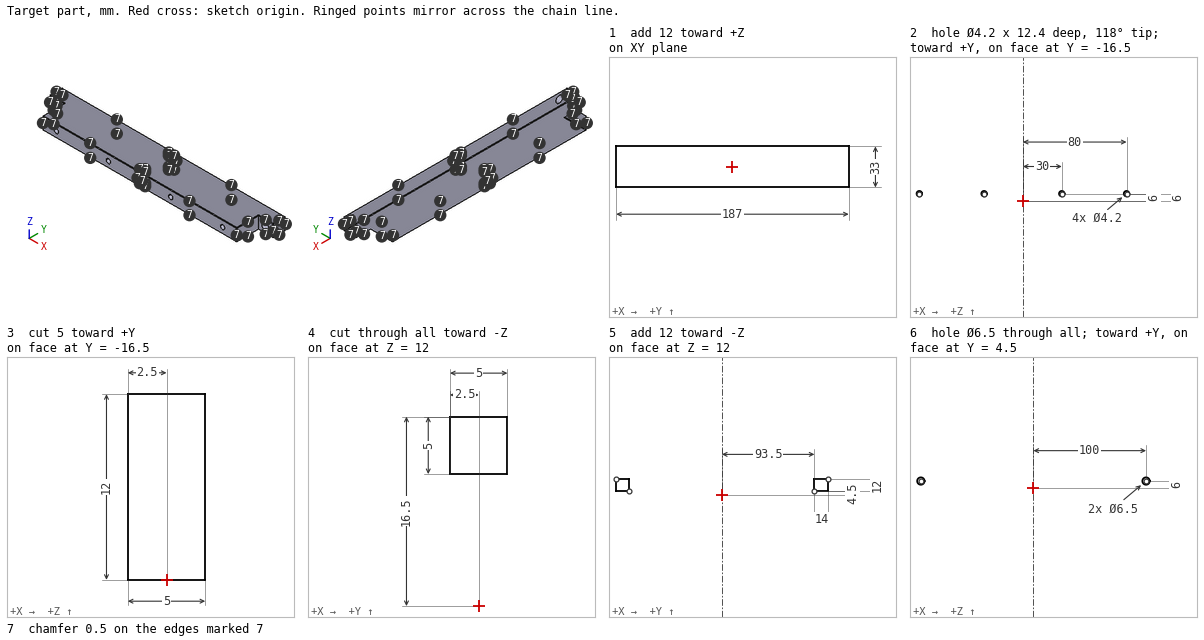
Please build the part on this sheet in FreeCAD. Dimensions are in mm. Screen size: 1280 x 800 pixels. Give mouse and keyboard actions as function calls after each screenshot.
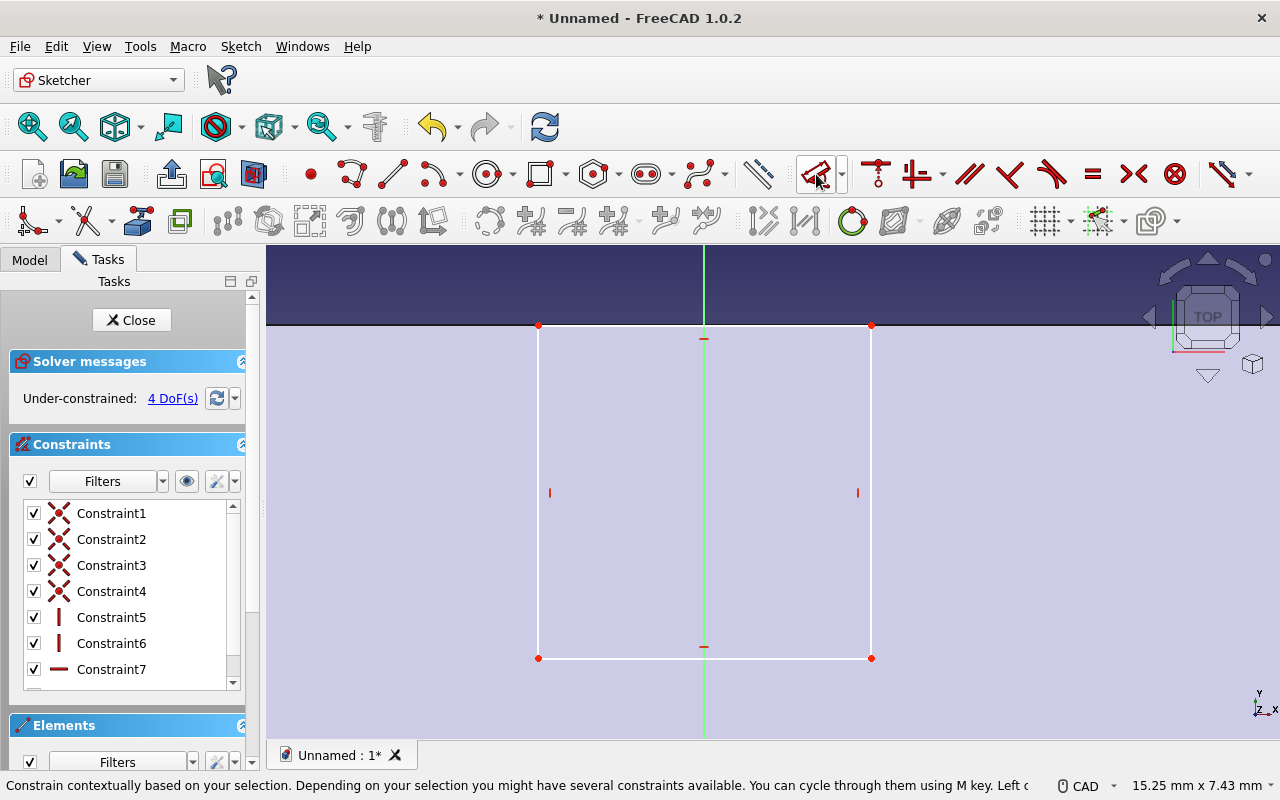
click(538, 426)
click(504, 493)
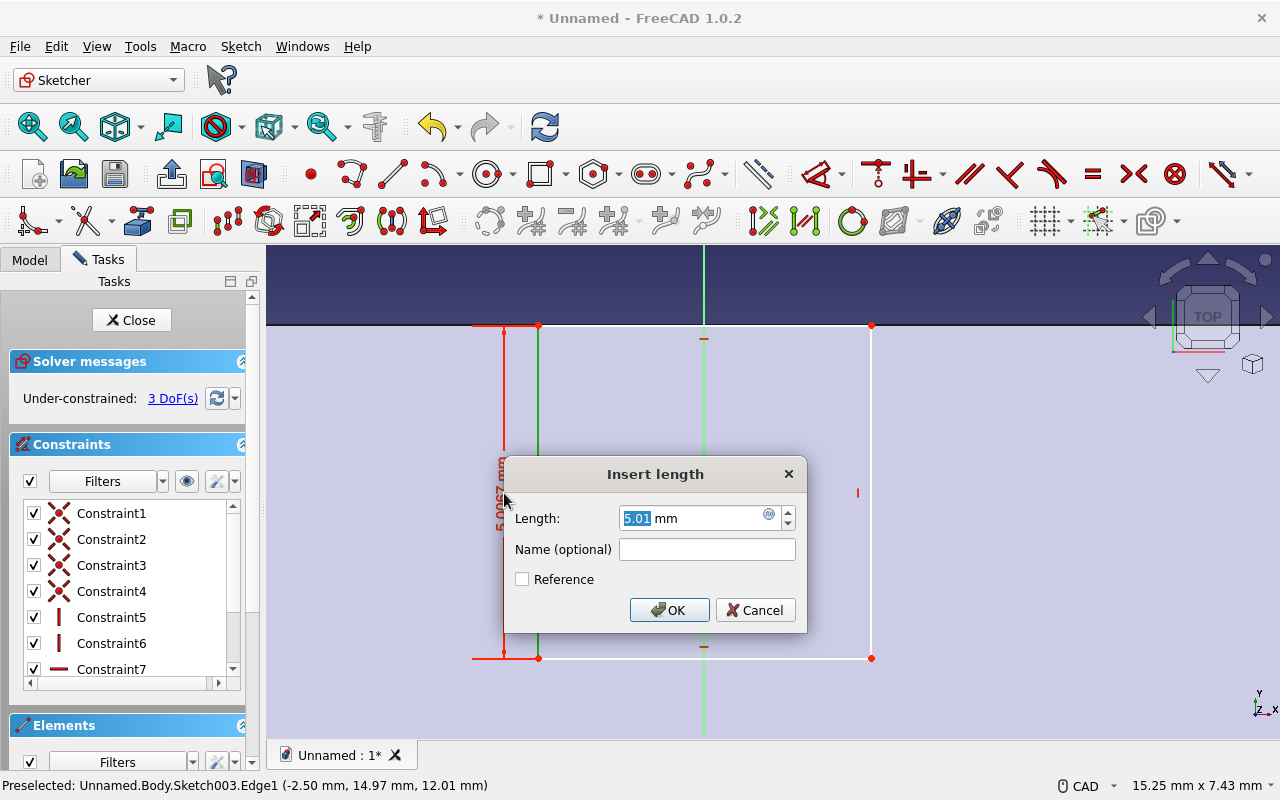
text(5)
key(Return)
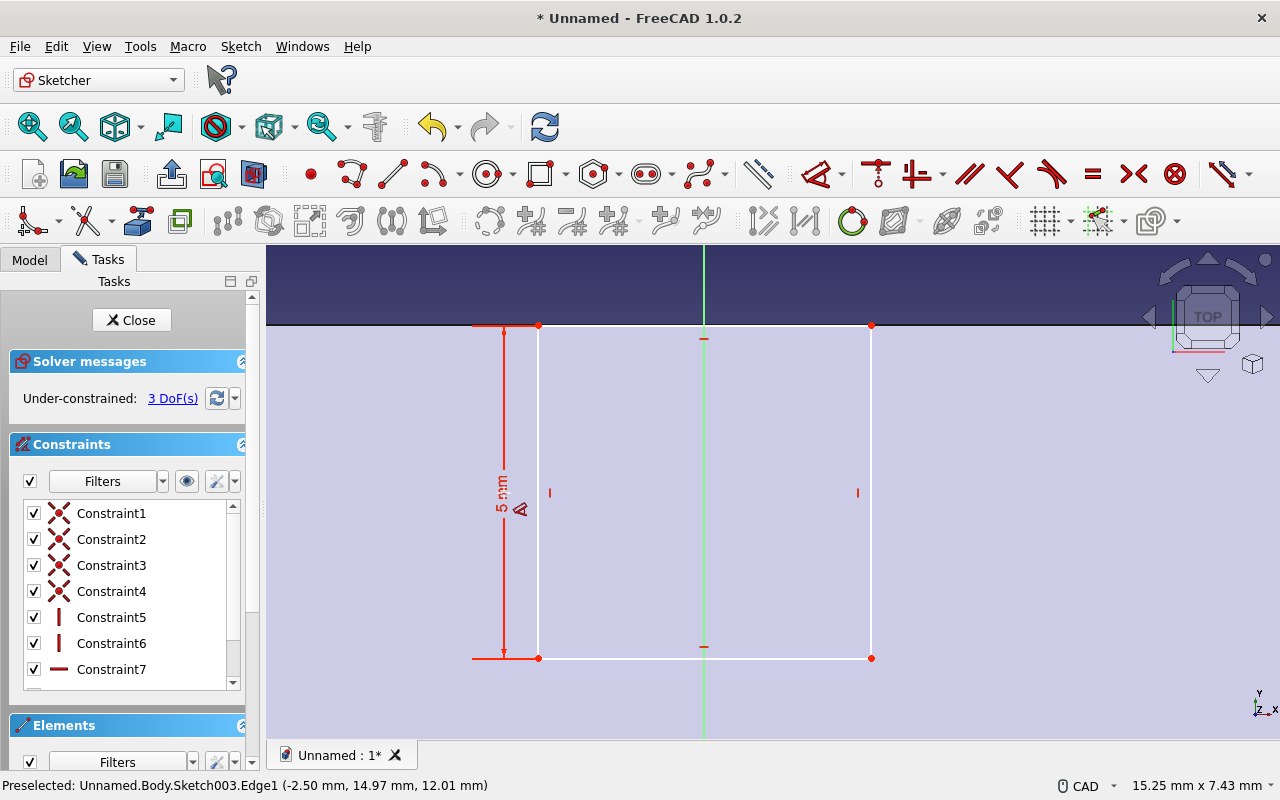
click(638, 659)
click(628, 693)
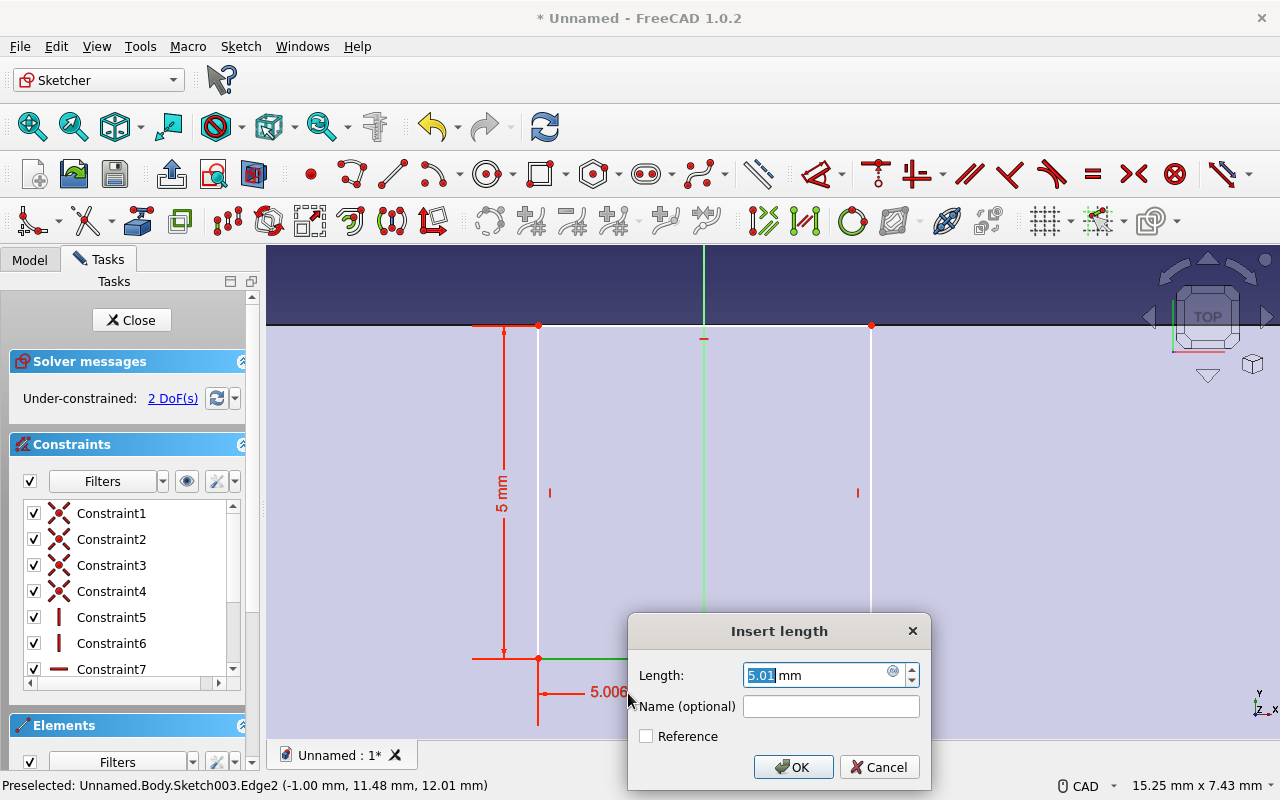
text(5)
key(Return)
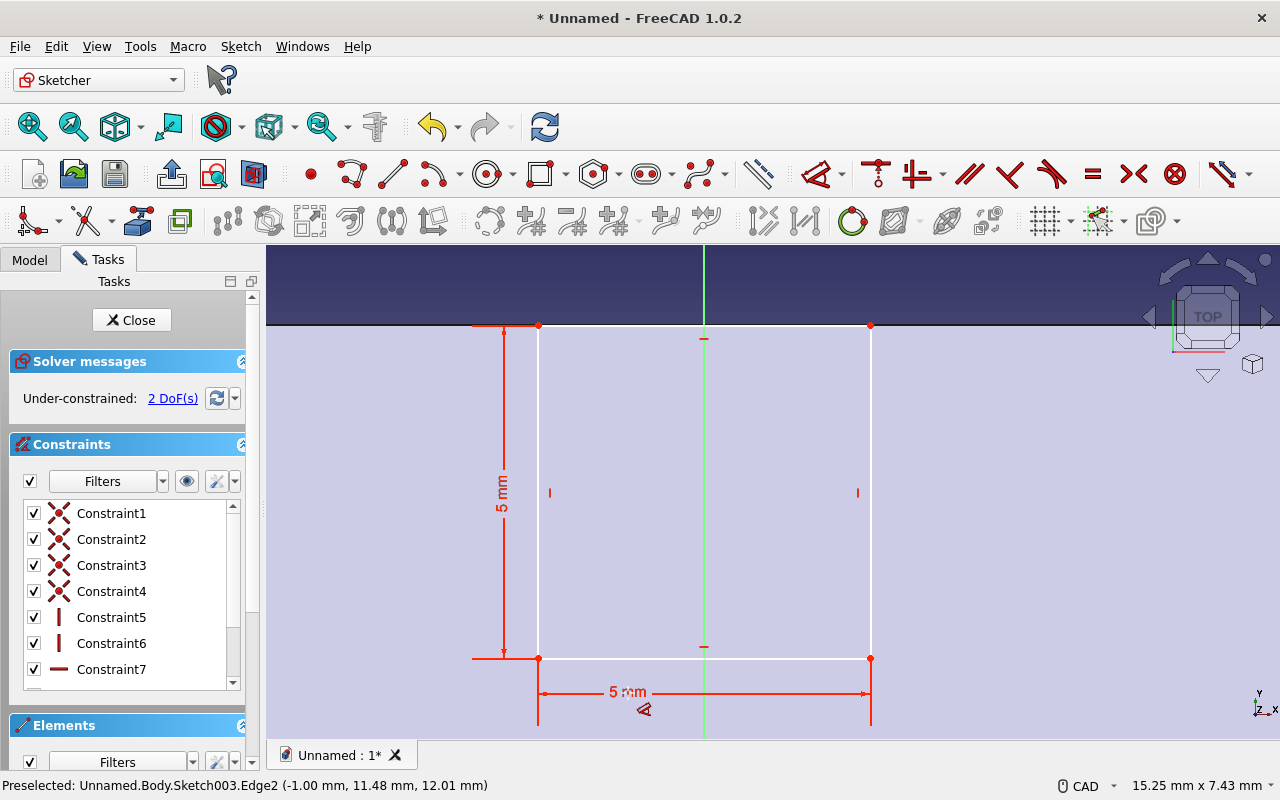
click(538, 326)
click(621, 292)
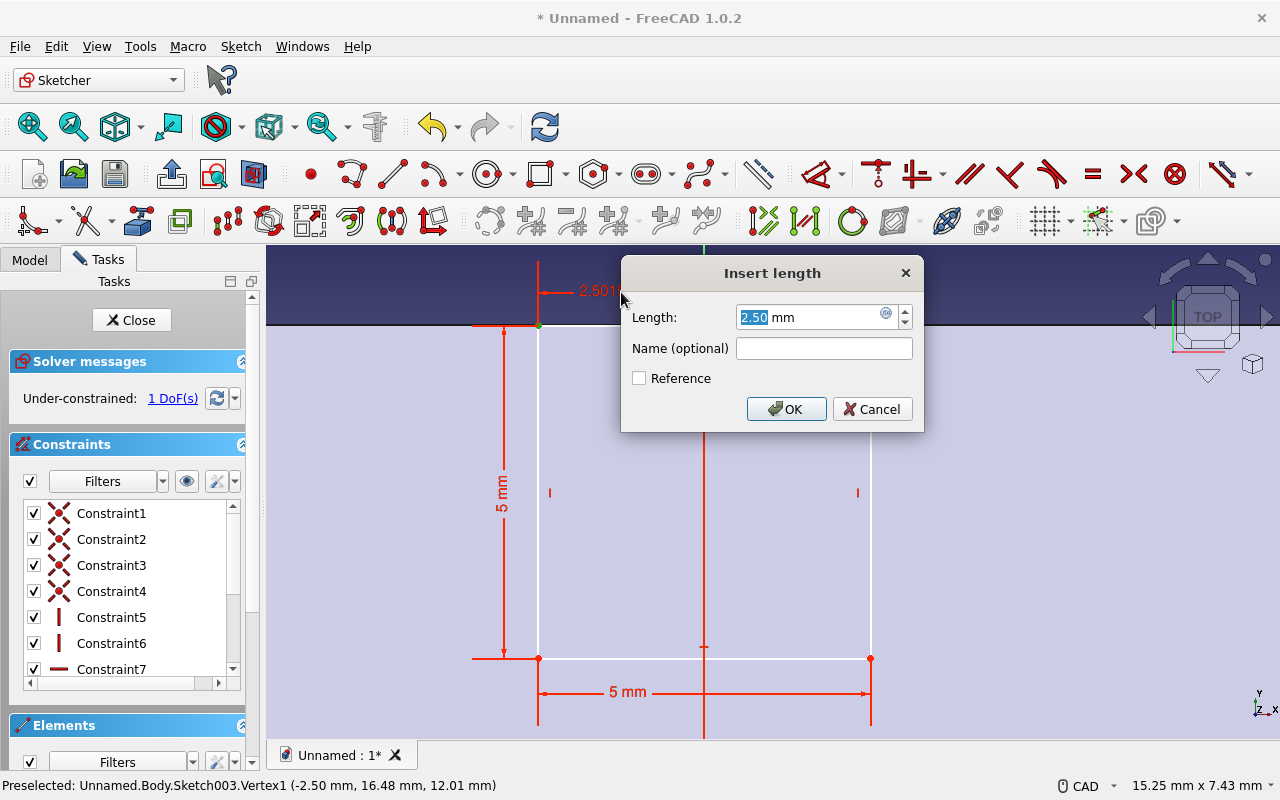
text(2.5)
key(Return)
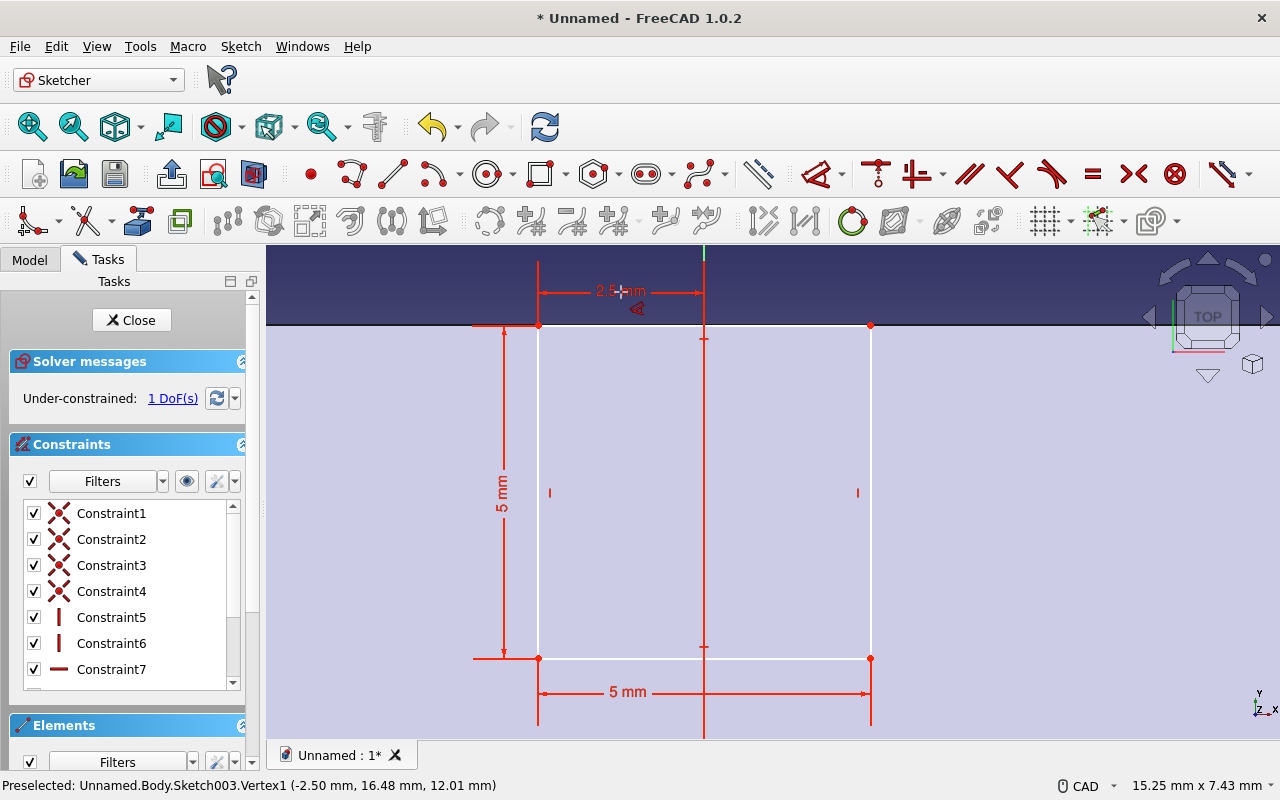
click(538, 326)
click(504, 519)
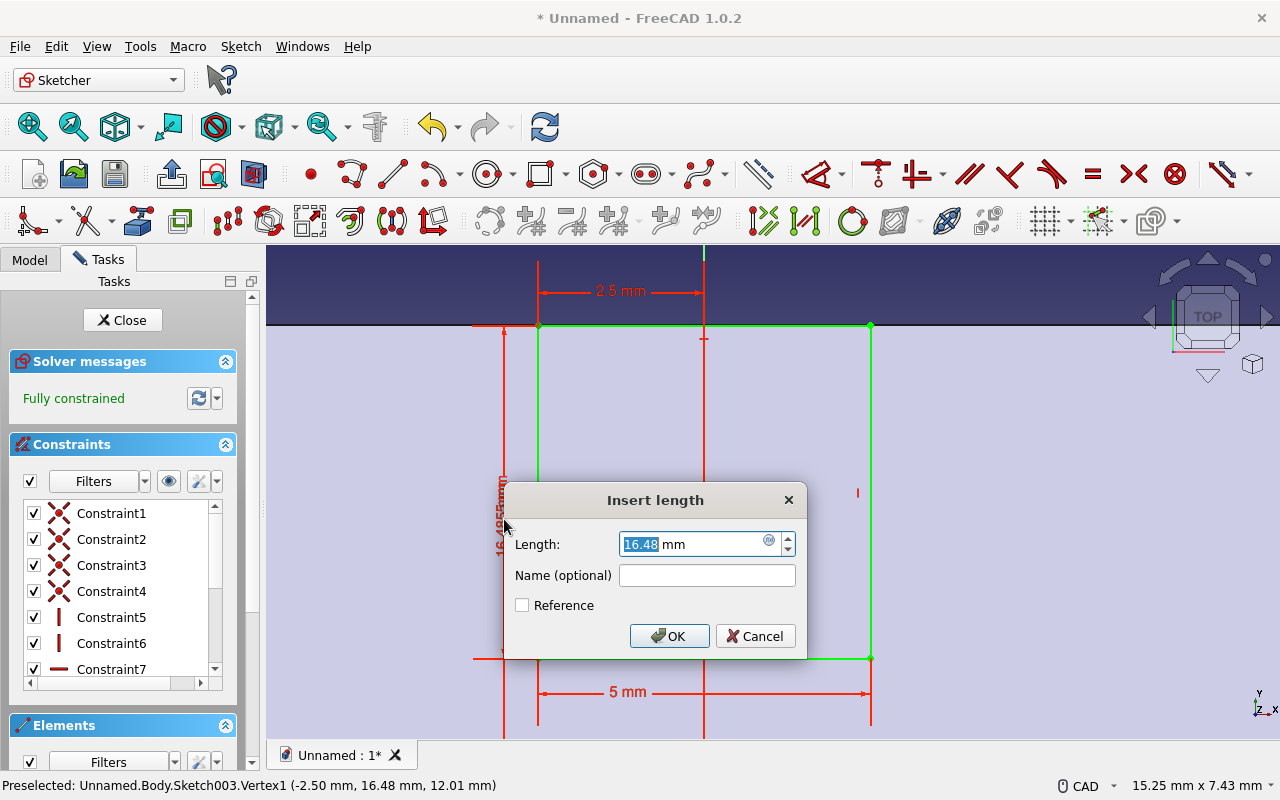
text(16.5)
key(Return)
key(Escape)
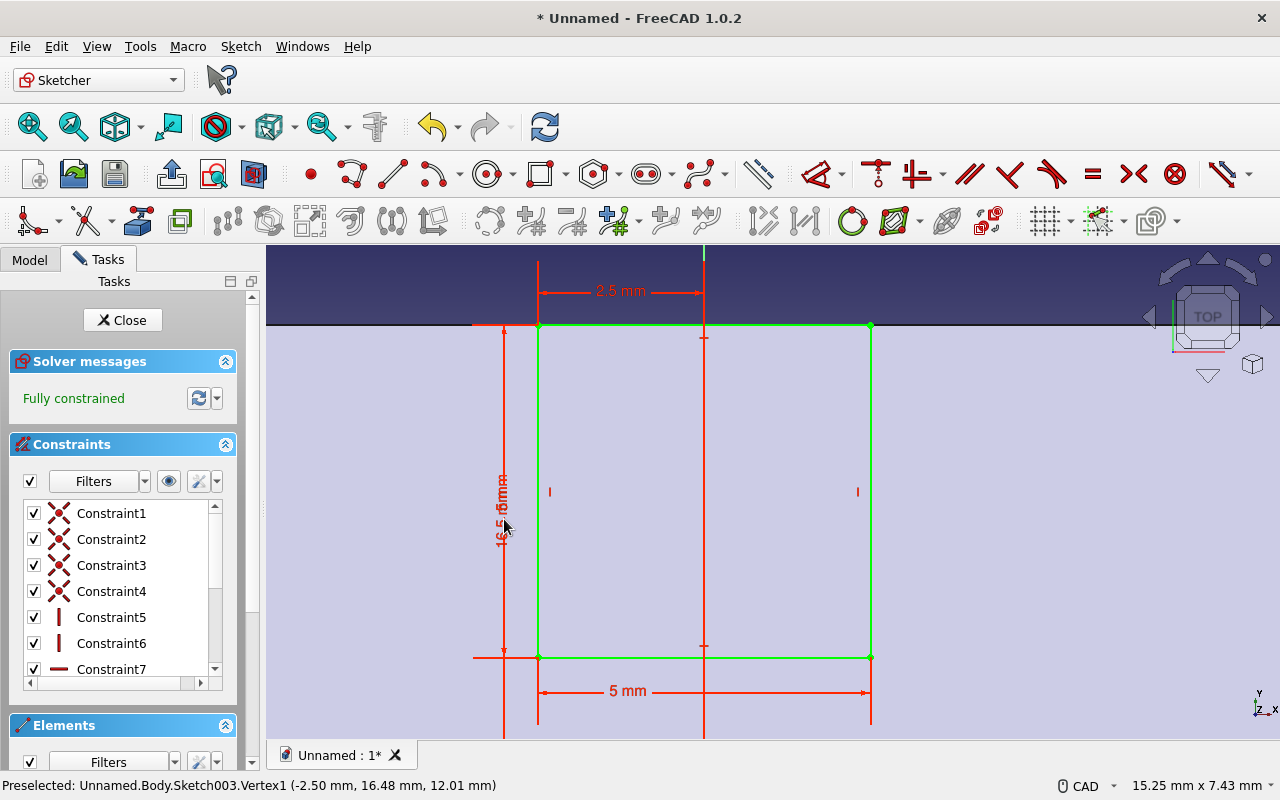
click(123, 320)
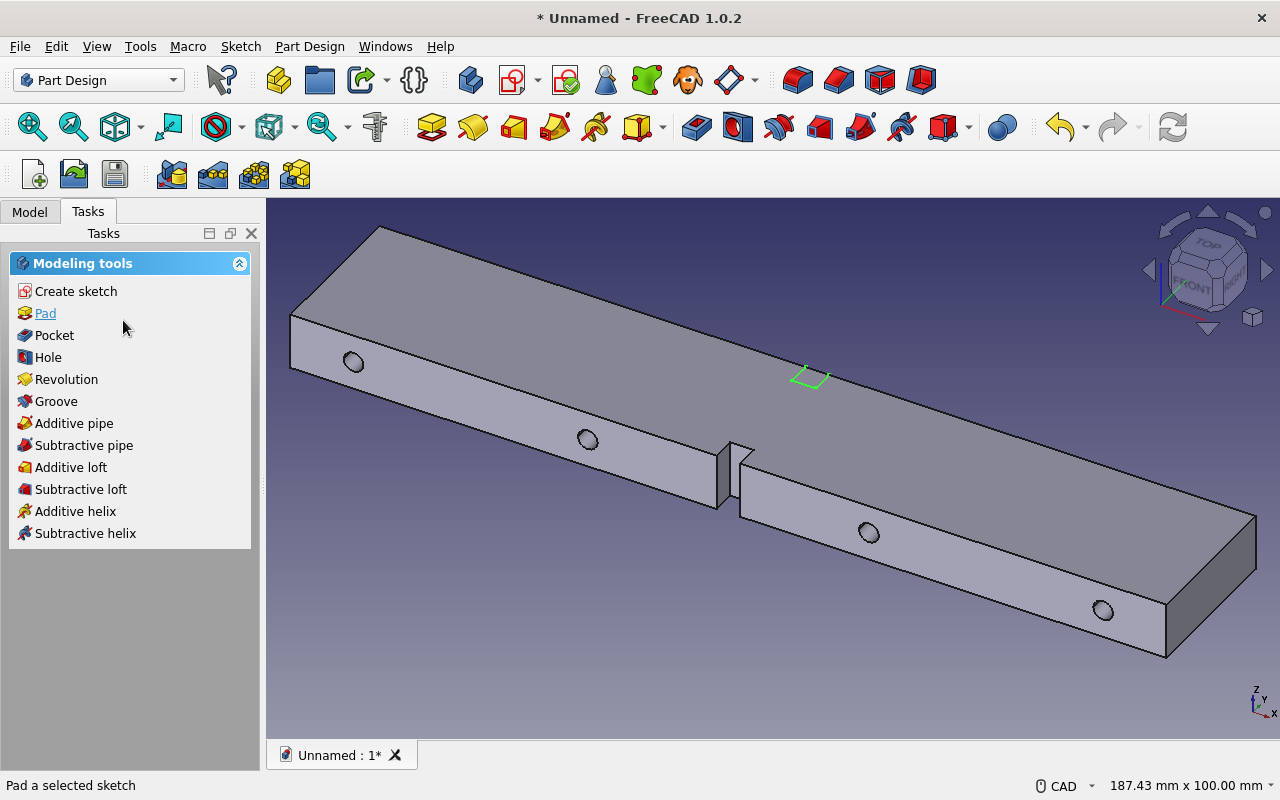
click(697, 128)